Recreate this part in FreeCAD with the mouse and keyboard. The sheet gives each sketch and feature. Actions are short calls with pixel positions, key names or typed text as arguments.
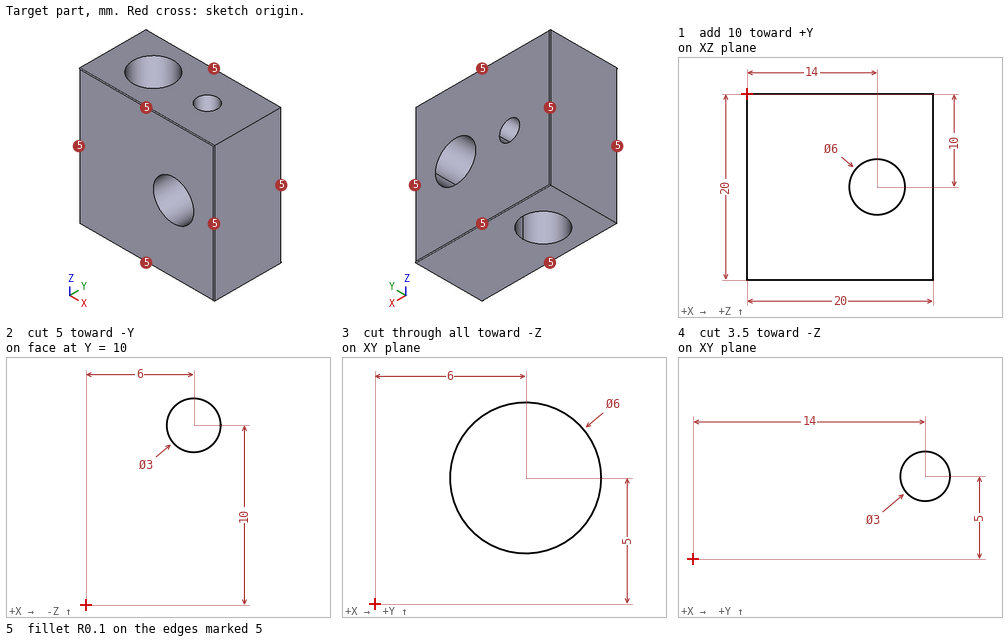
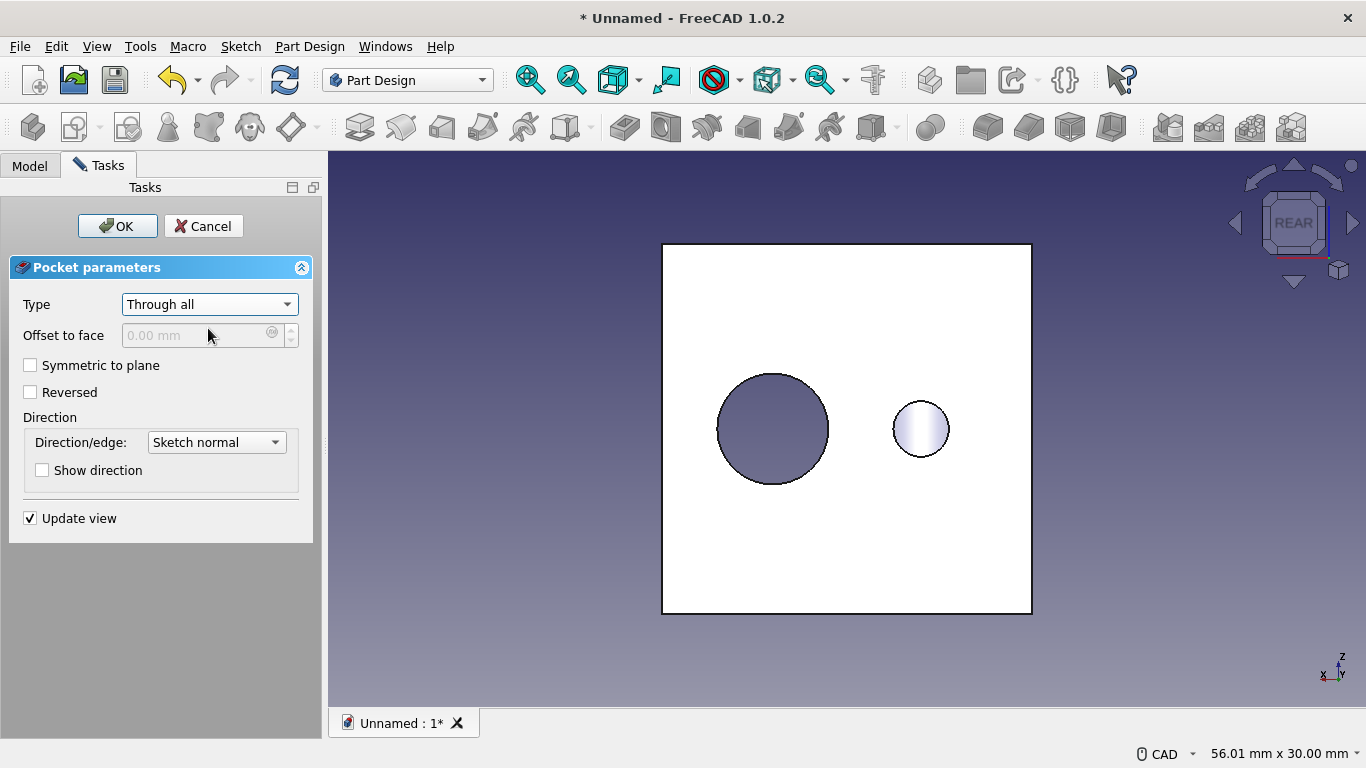
click(118, 226)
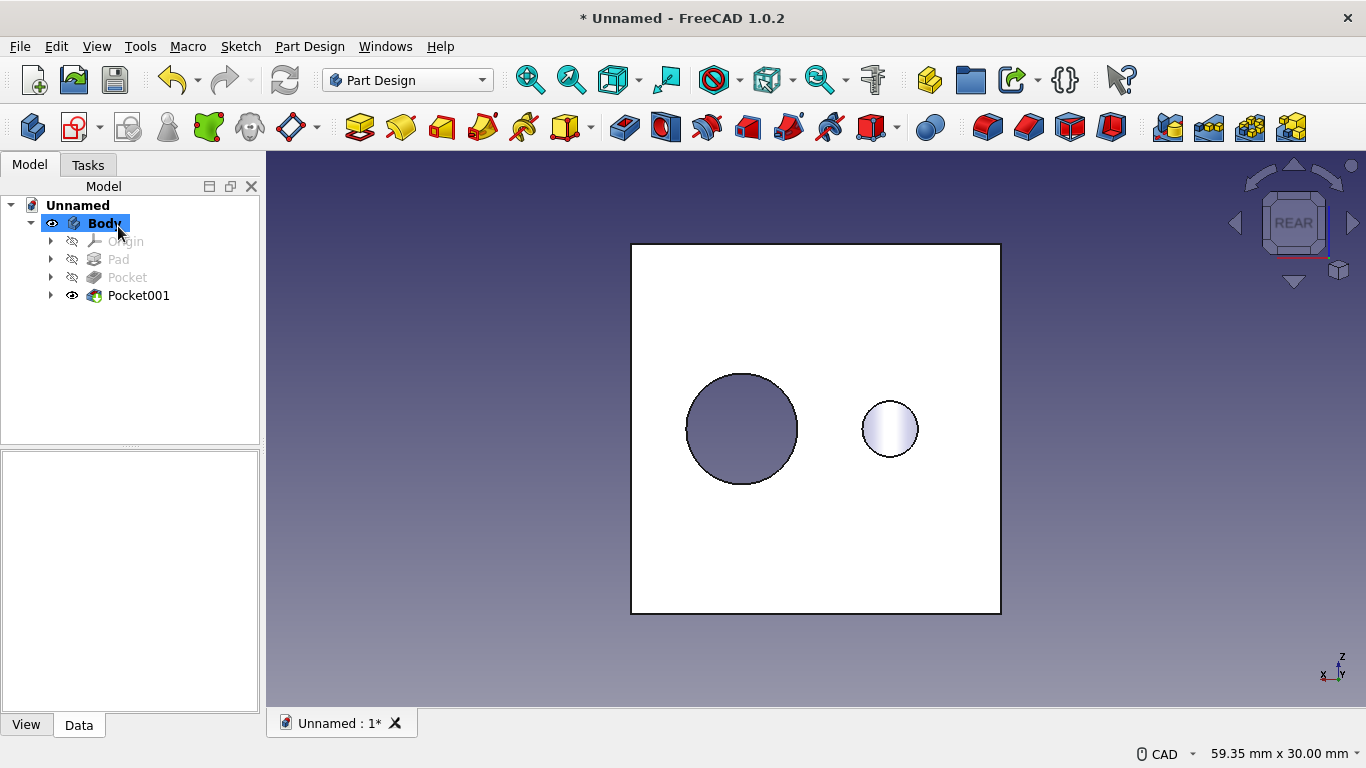
click(74, 128)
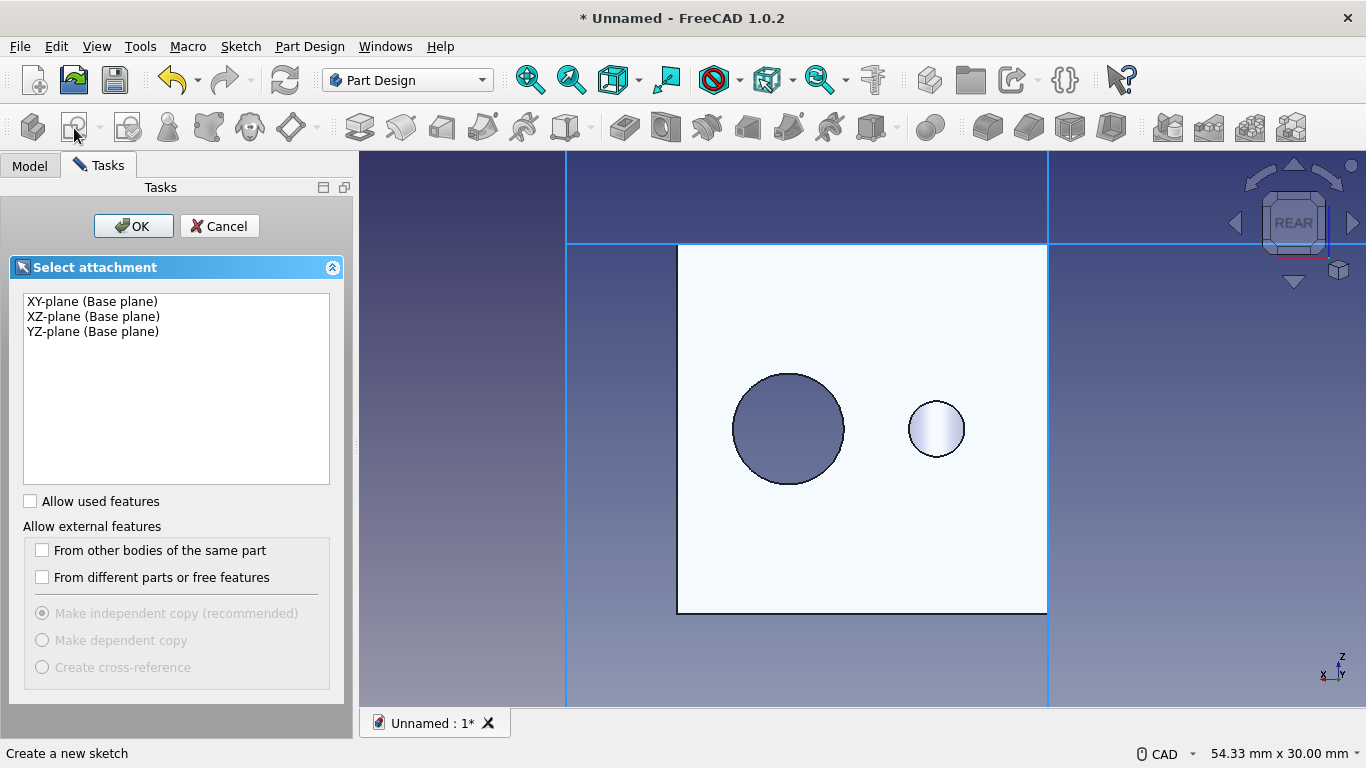
click(84, 302)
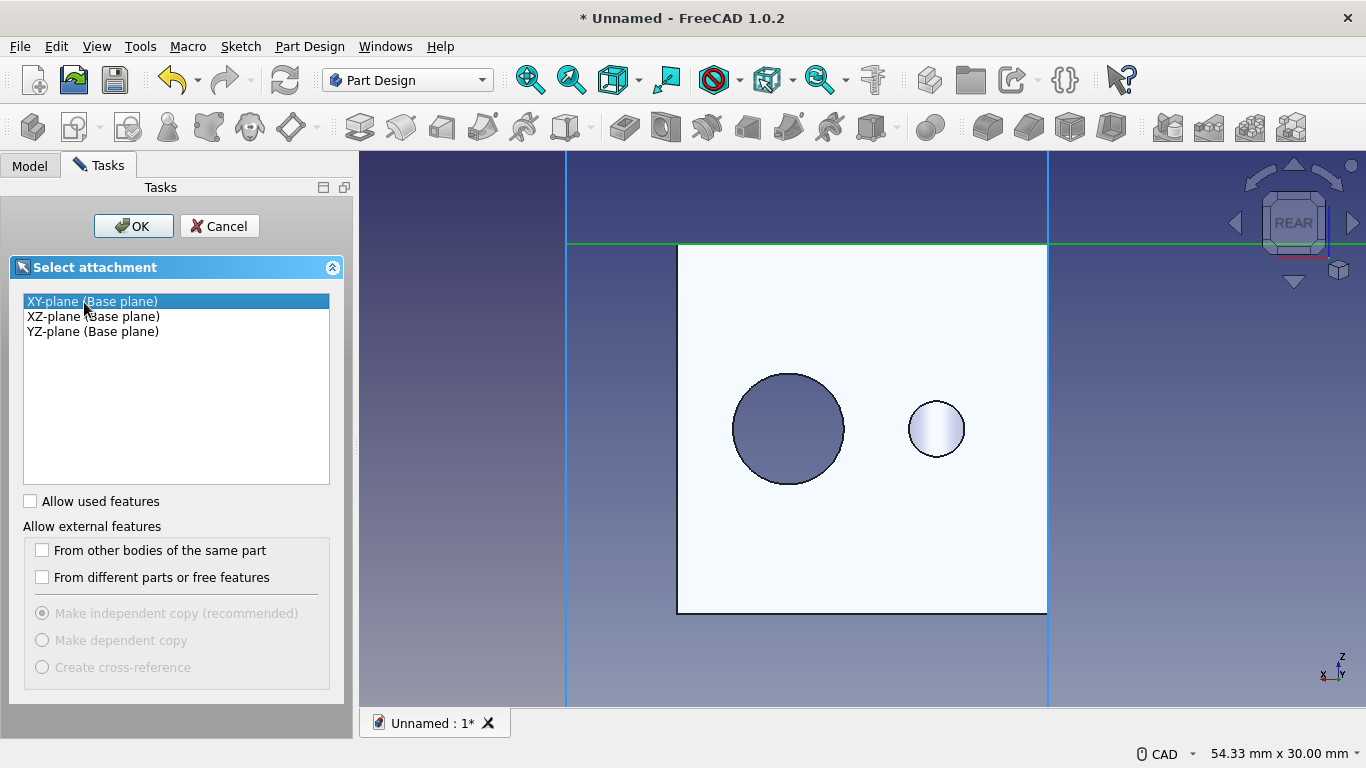
click(134, 226)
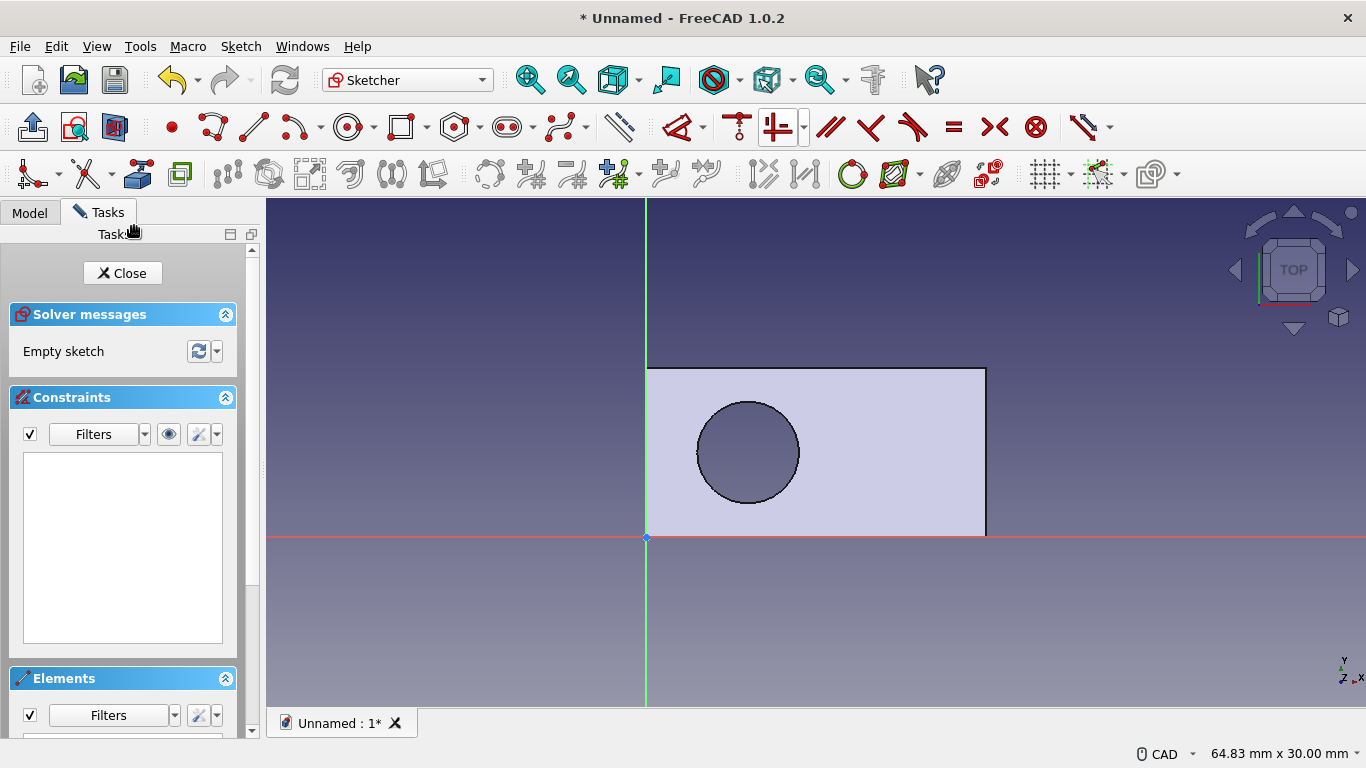
scroll(911, 453, up, 9)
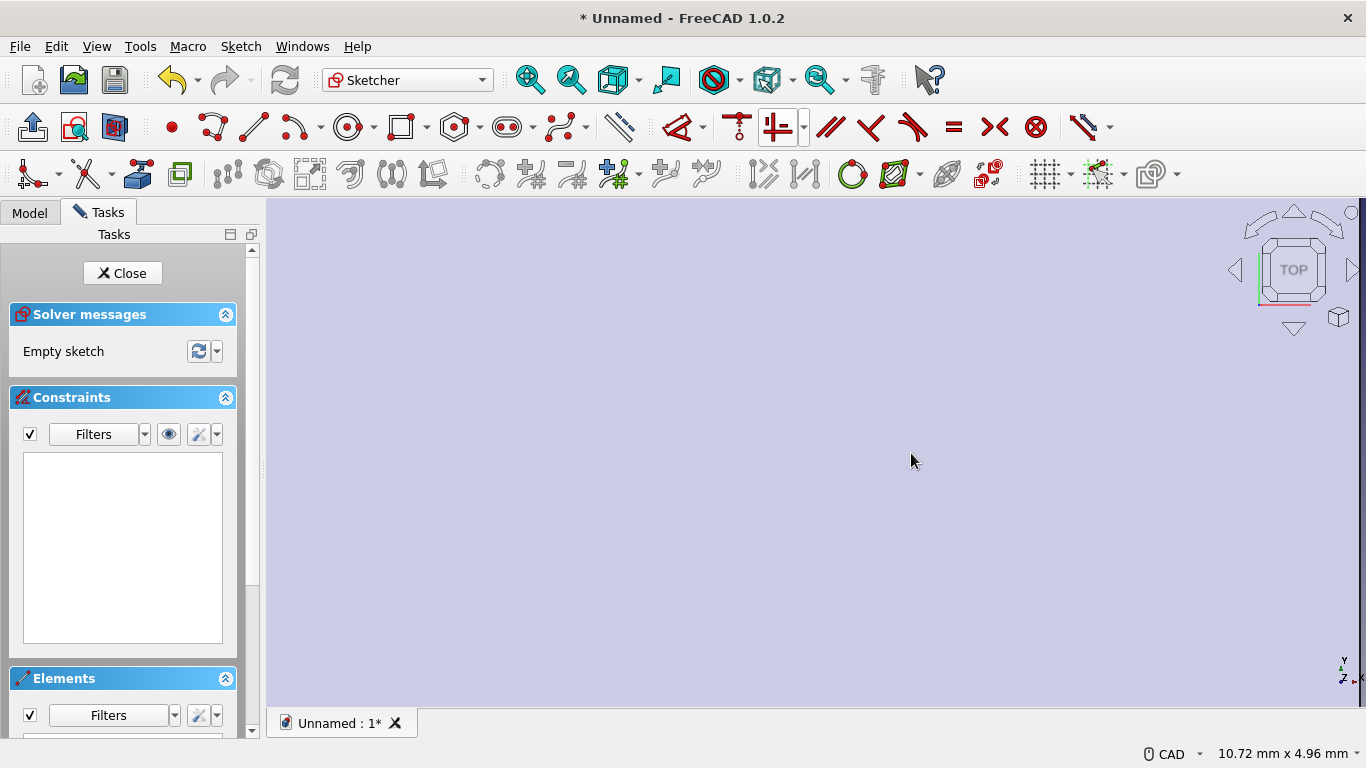
click(348, 128)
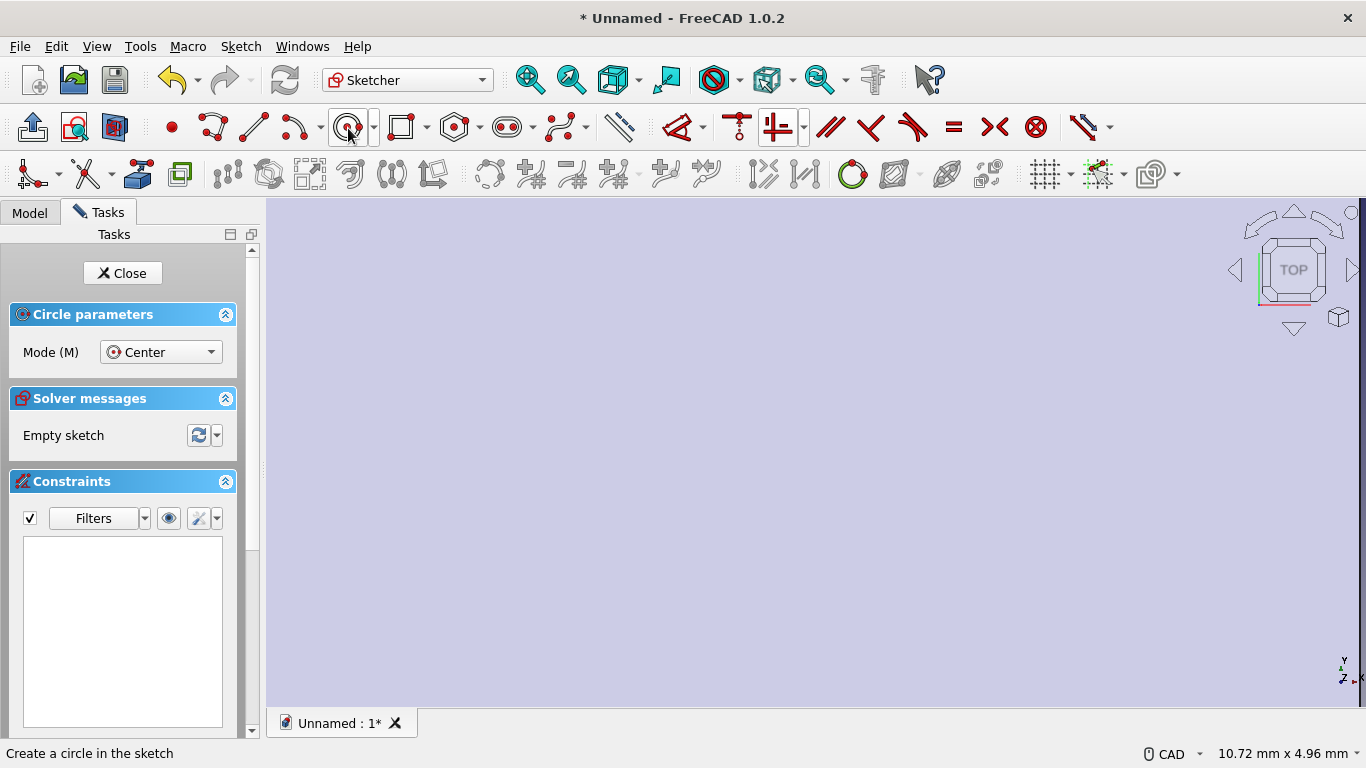
click(744, 447)
click(853, 339)
key(Escape)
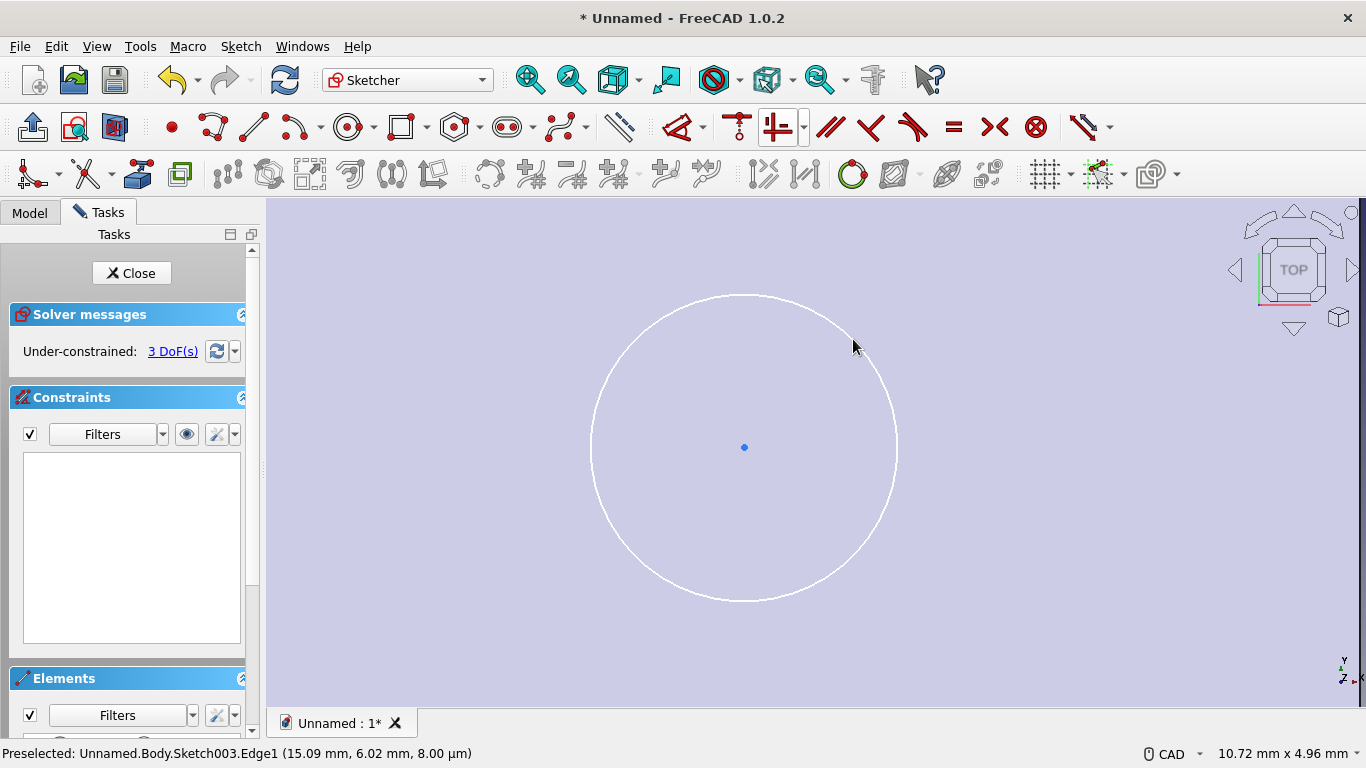
click(676, 128)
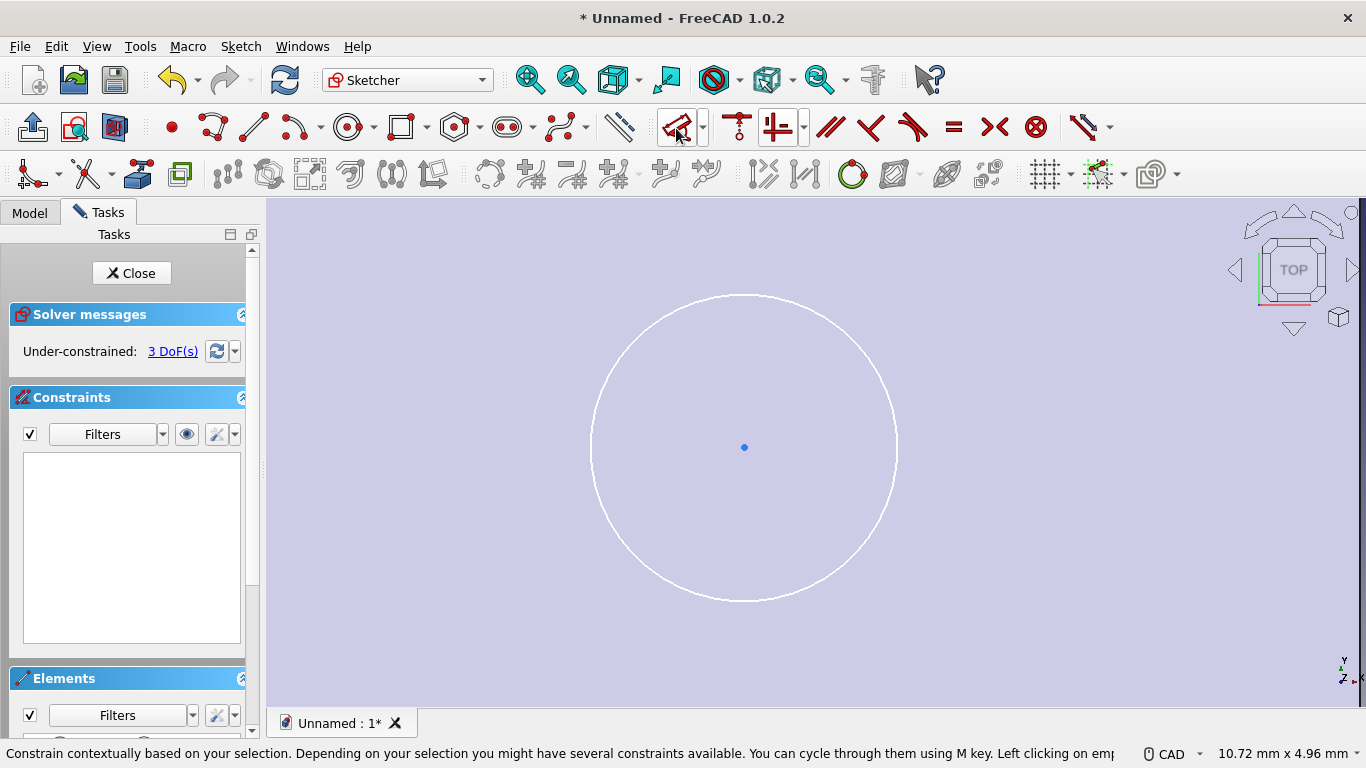
click(852, 339)
click(875, 316)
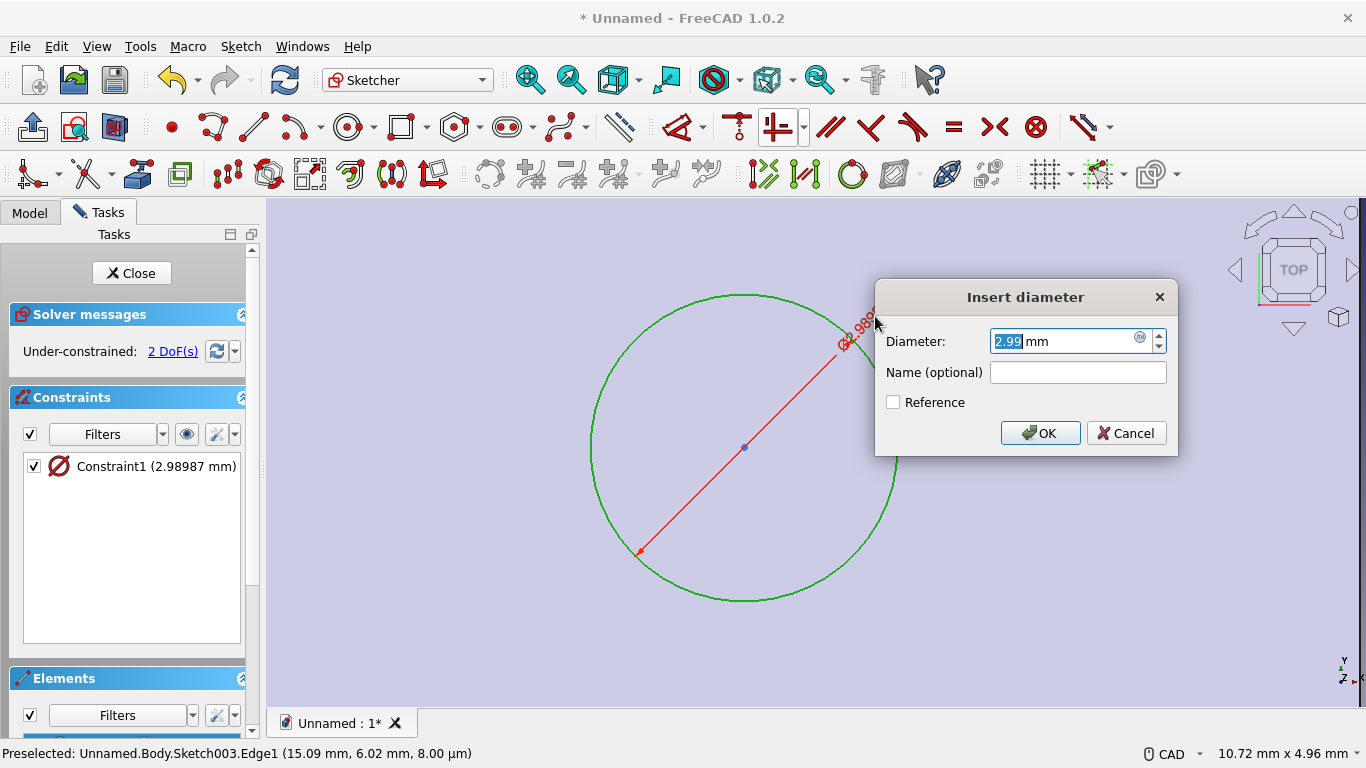
text(3)
key(Return)